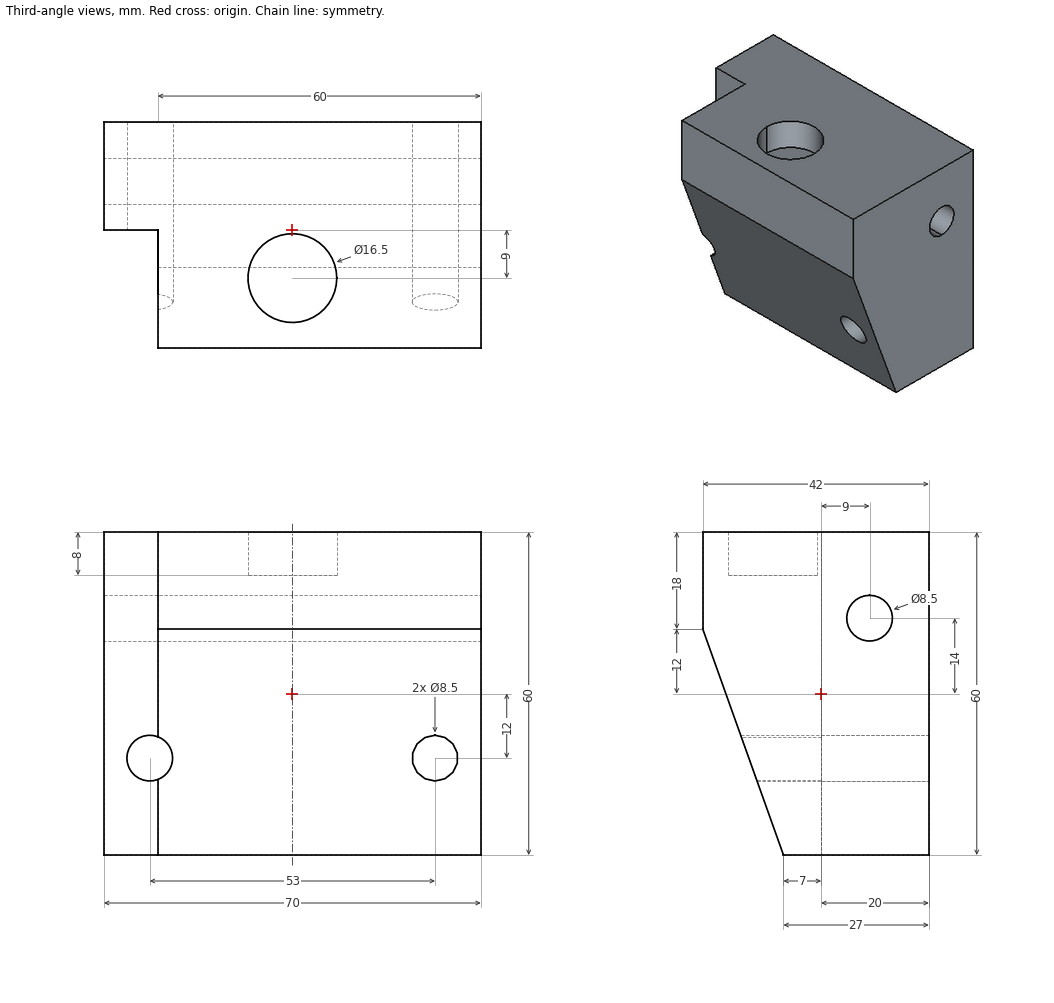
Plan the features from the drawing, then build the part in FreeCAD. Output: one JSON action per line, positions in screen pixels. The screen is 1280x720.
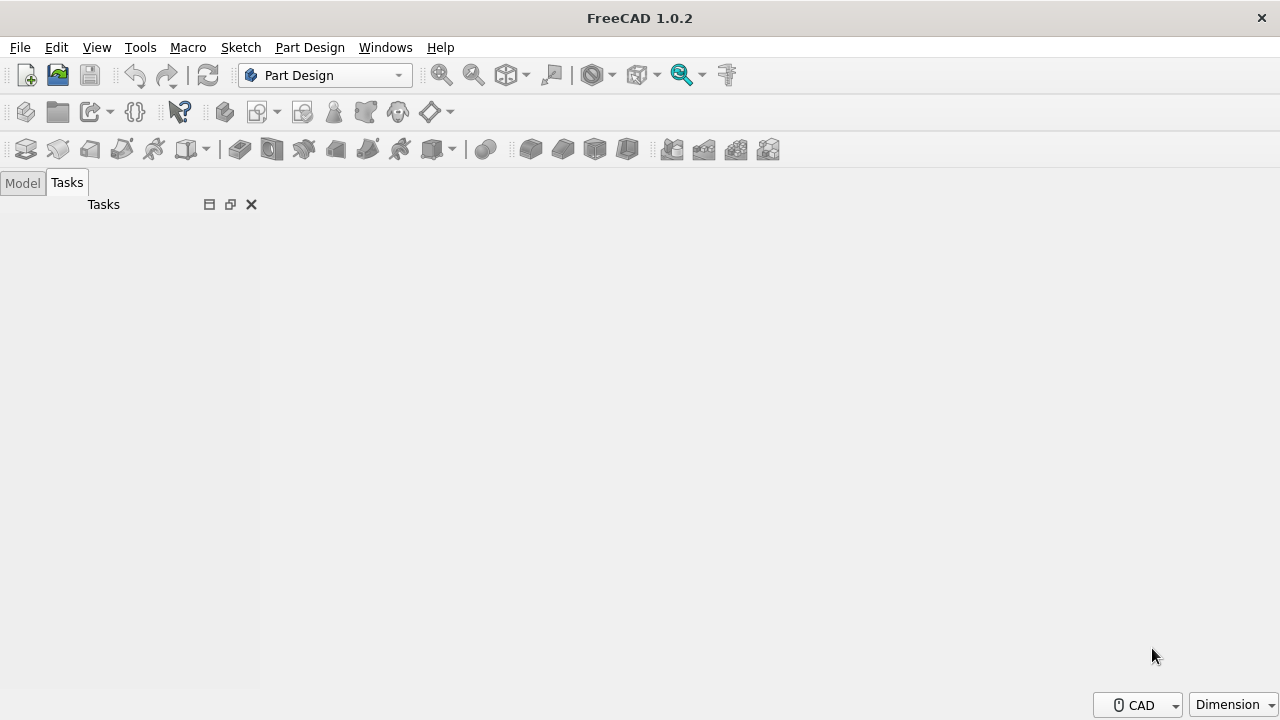
{"action": "key", "text": "ctrl+n"}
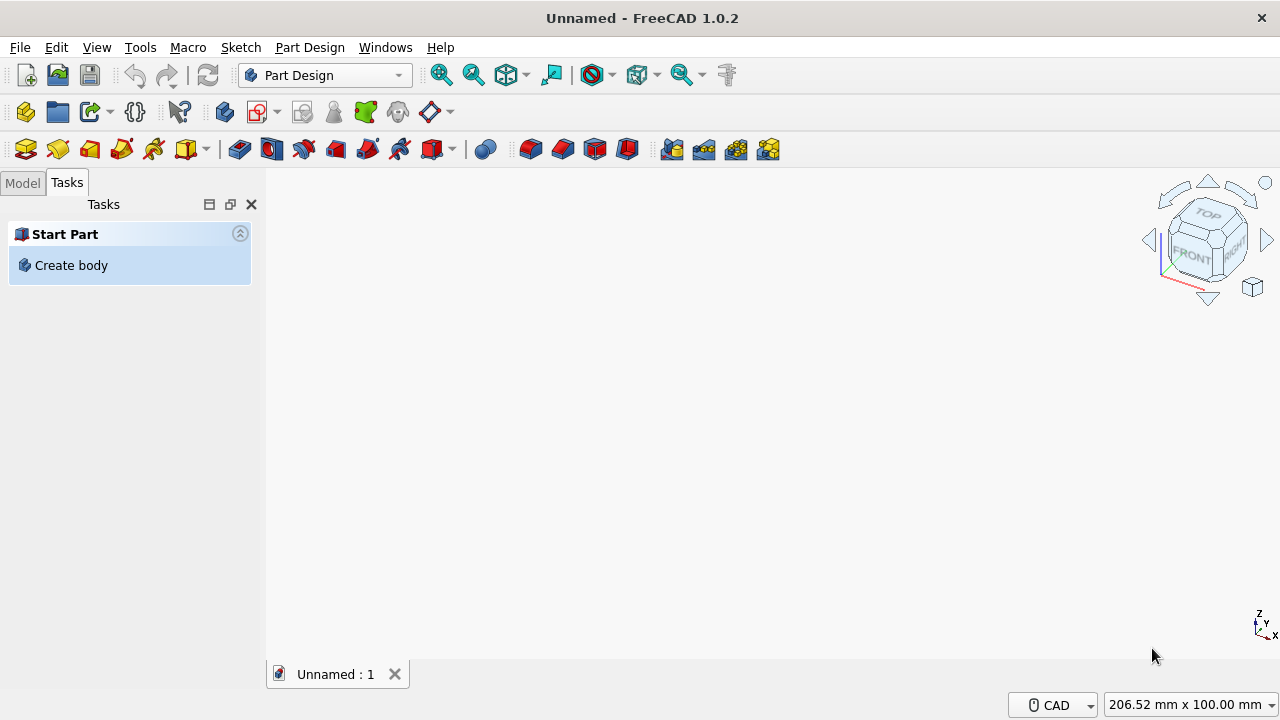
{"action": "left_click", "coordinate": [258, 112]}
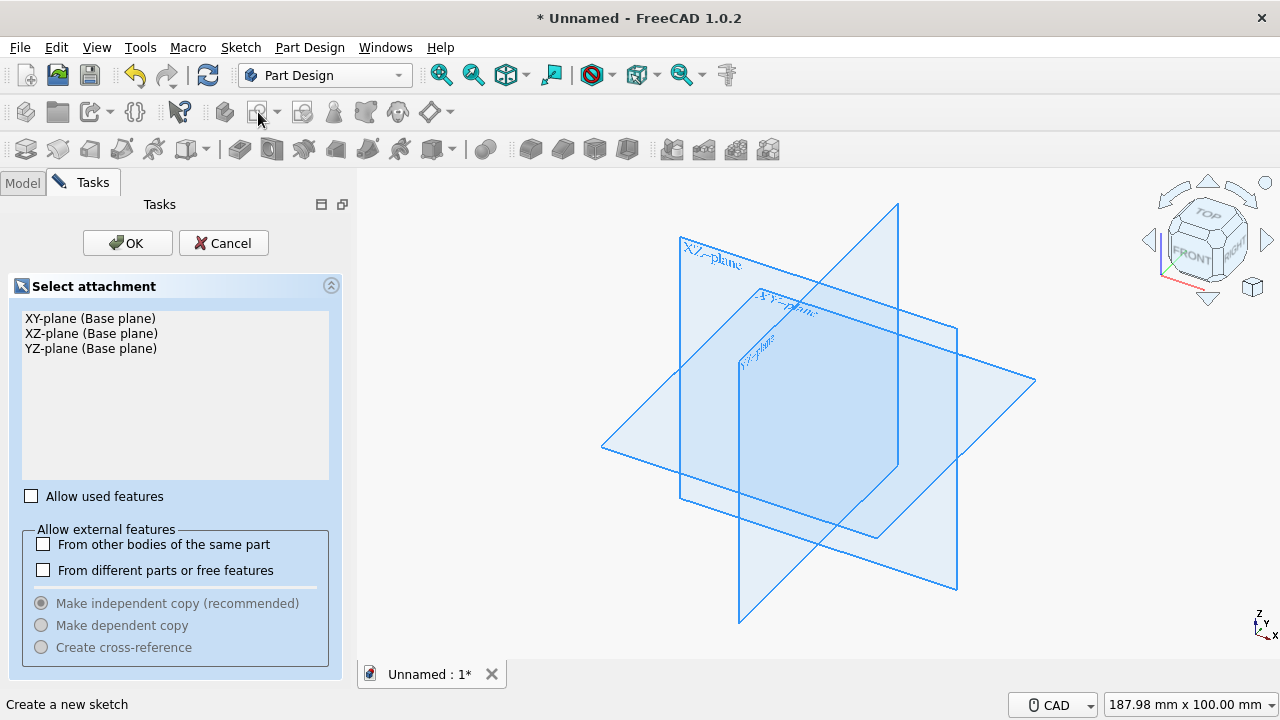
{"action": "left_click", "coordinate": [82, 334]}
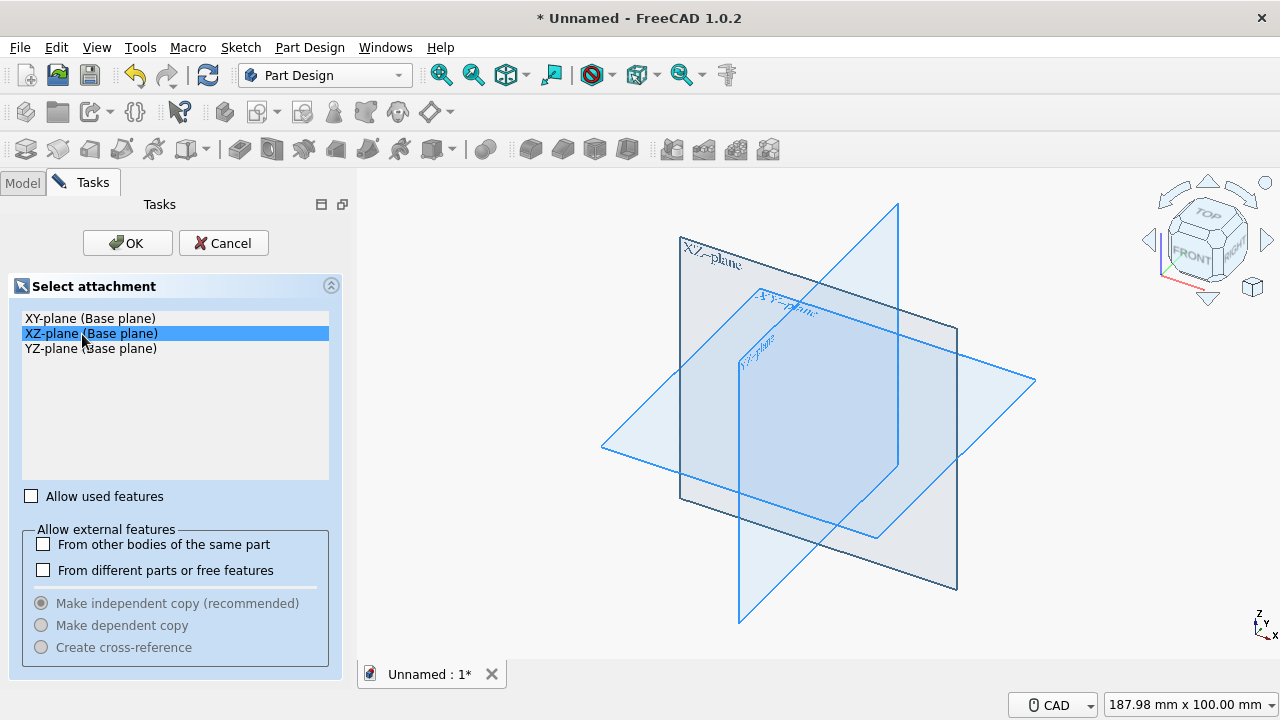
{"action": "left_click", "coordinate": [128, 243]}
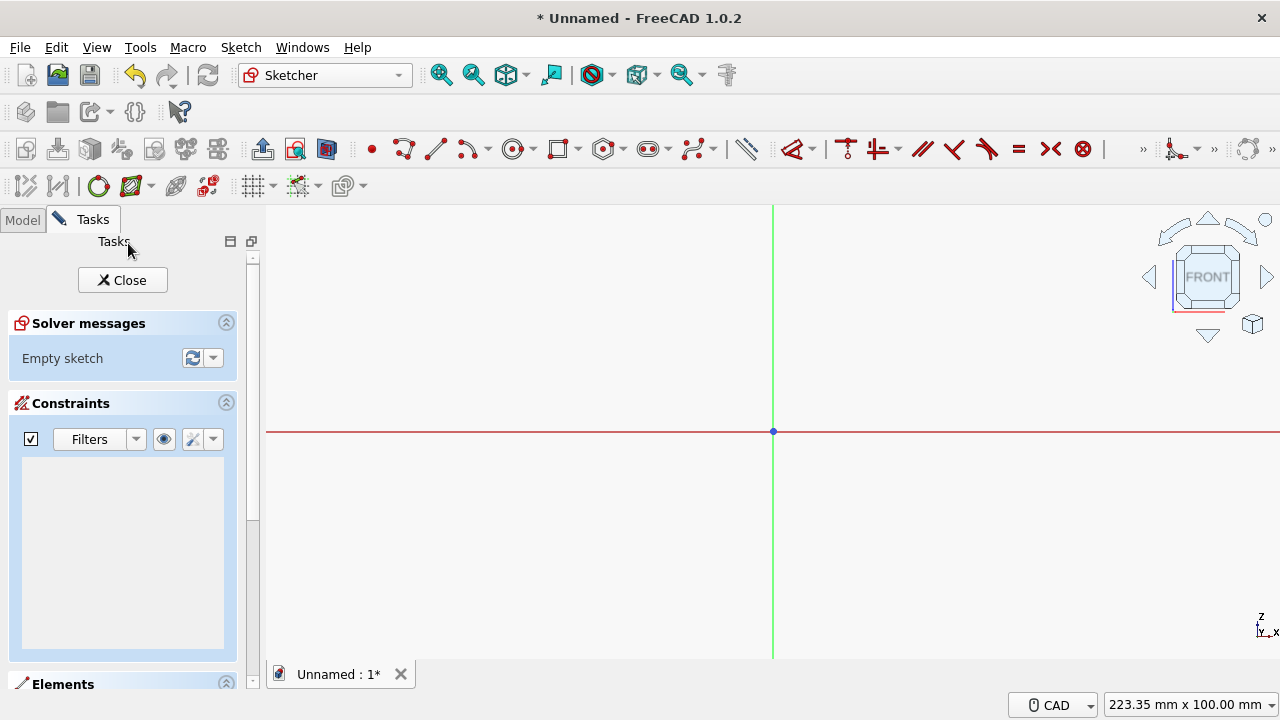
{"action": "left_click", "coordinate": [580, 150]}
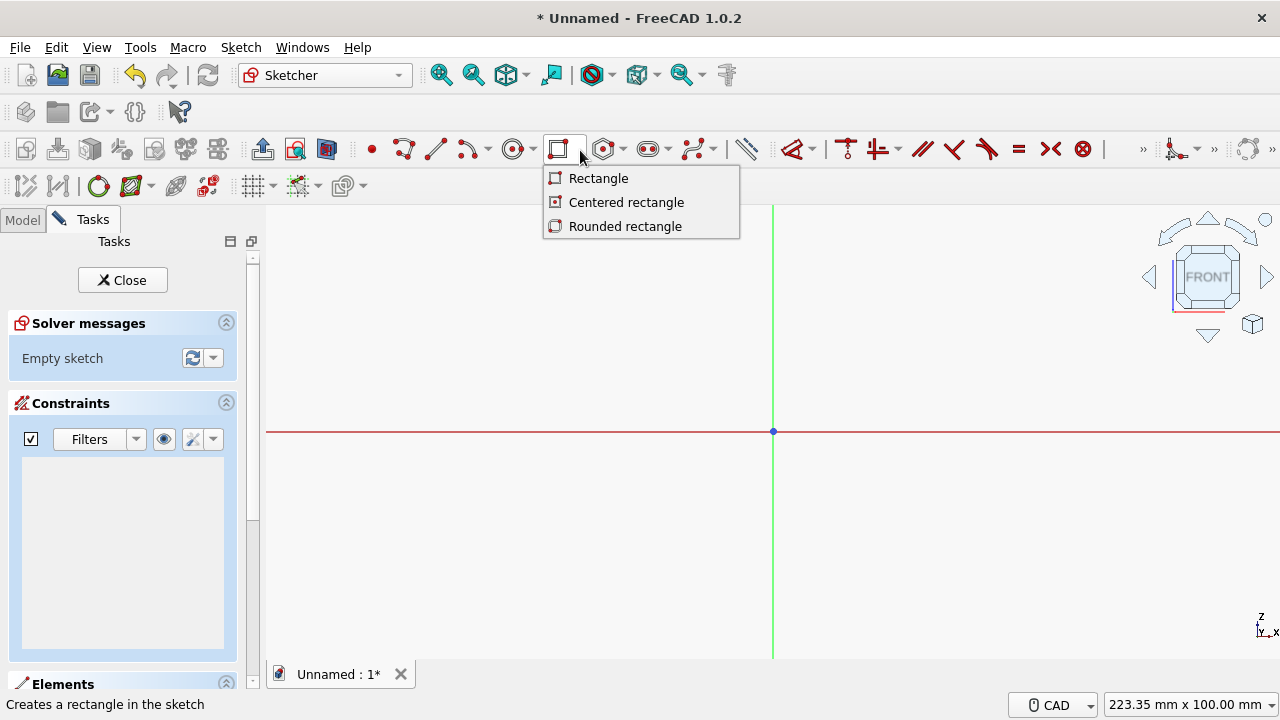
{"action": "left_click", "coordinate": [642, 202]}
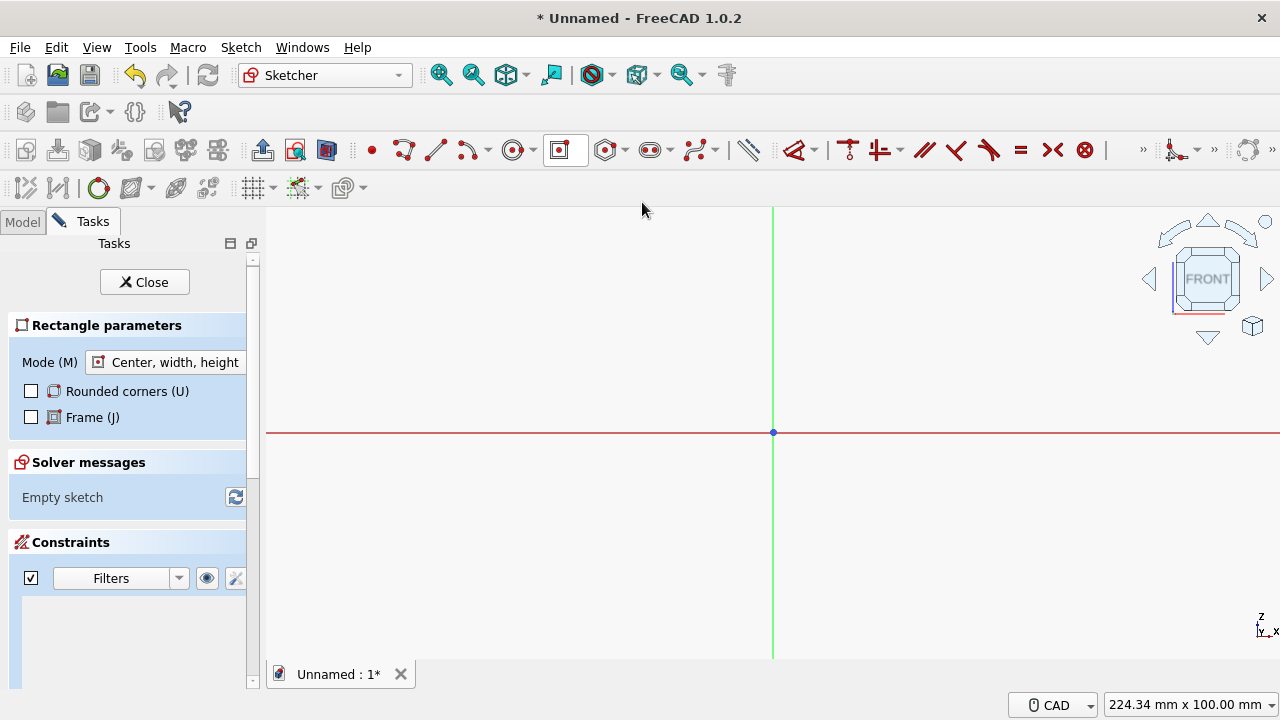
{"action": "left_click", "coordinate": [773, 433]}
{"action": "mouse_move", "coordinate": [931, 297]}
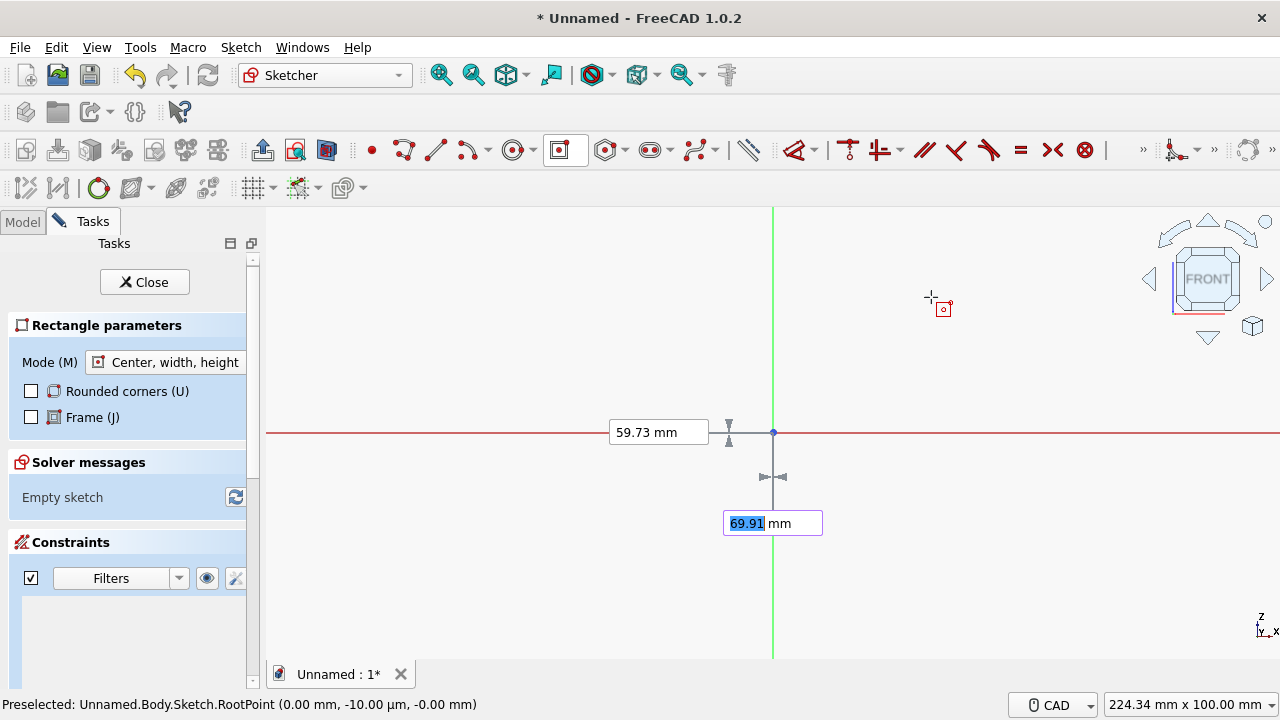
{"action": "type", "text": "70"}
{"action": "key", "text": "Tab"}
{"action": "type", "text": "60"}
{"action": "key", "text": "Return"}
{"action": "key", "text": "Escape"}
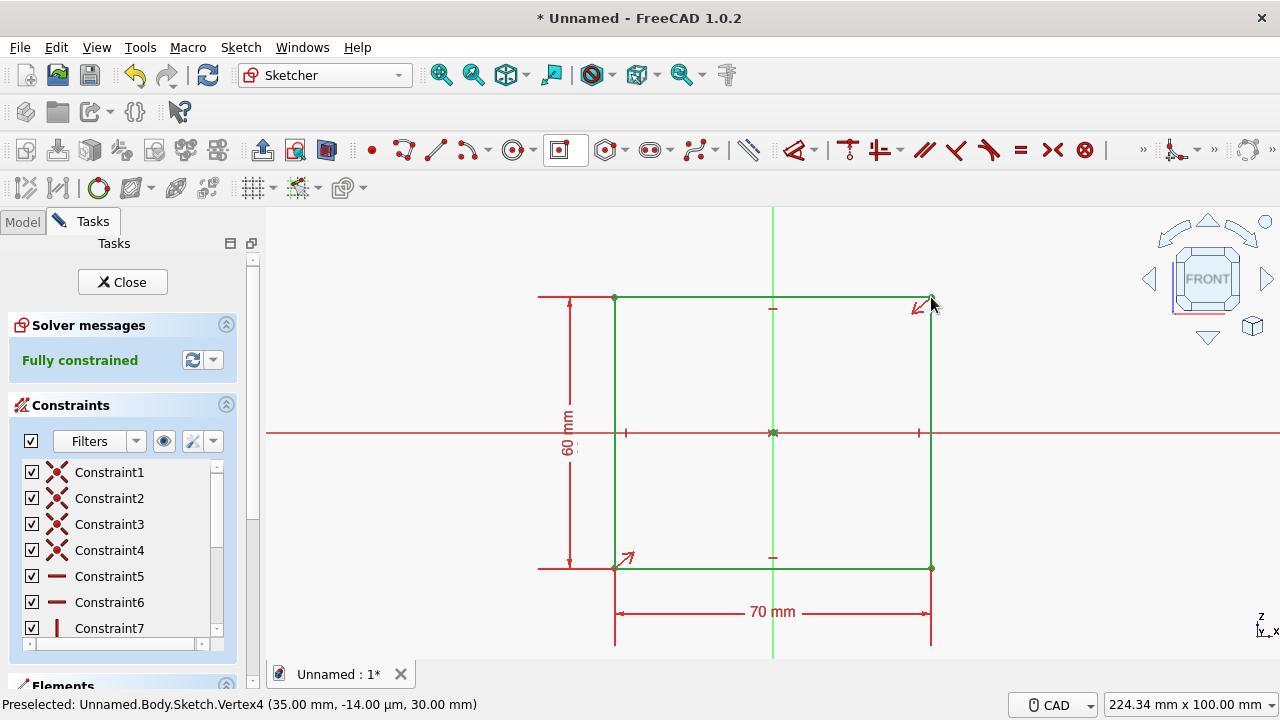
{"action": "left_click", "coordinate": [123, 282]}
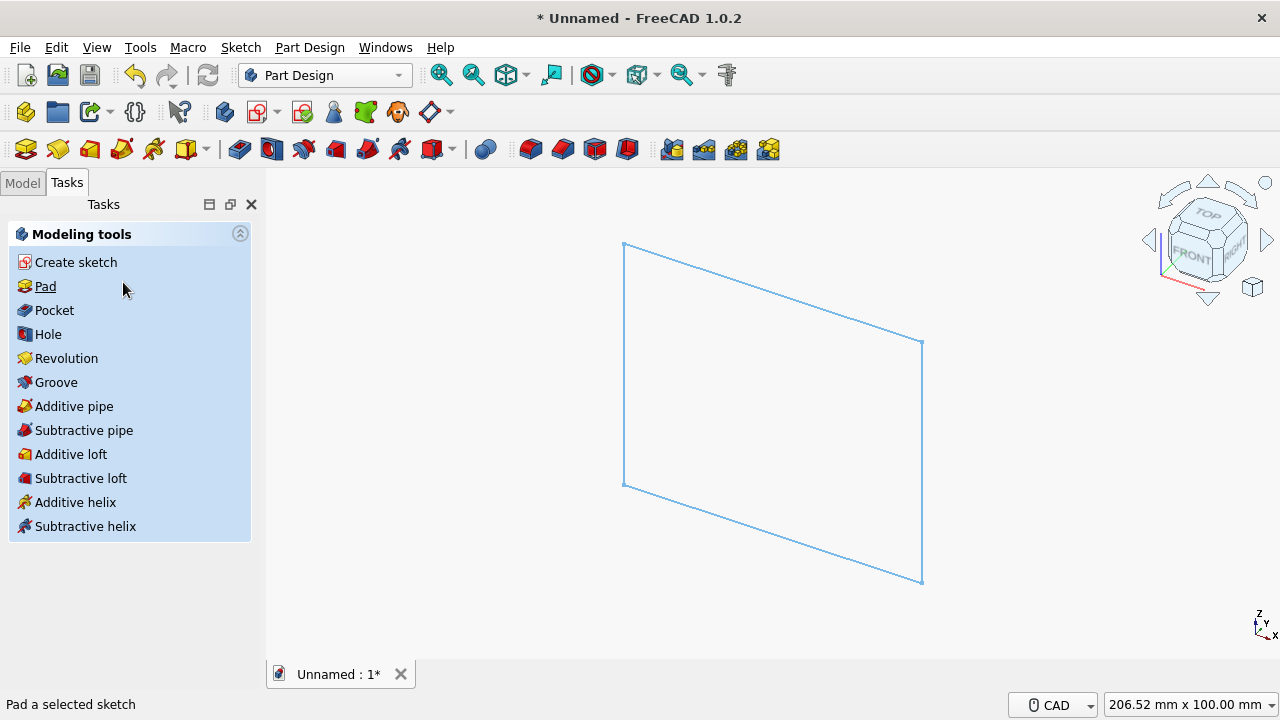
{"action": "left_click", "coordinate": [26, 150]}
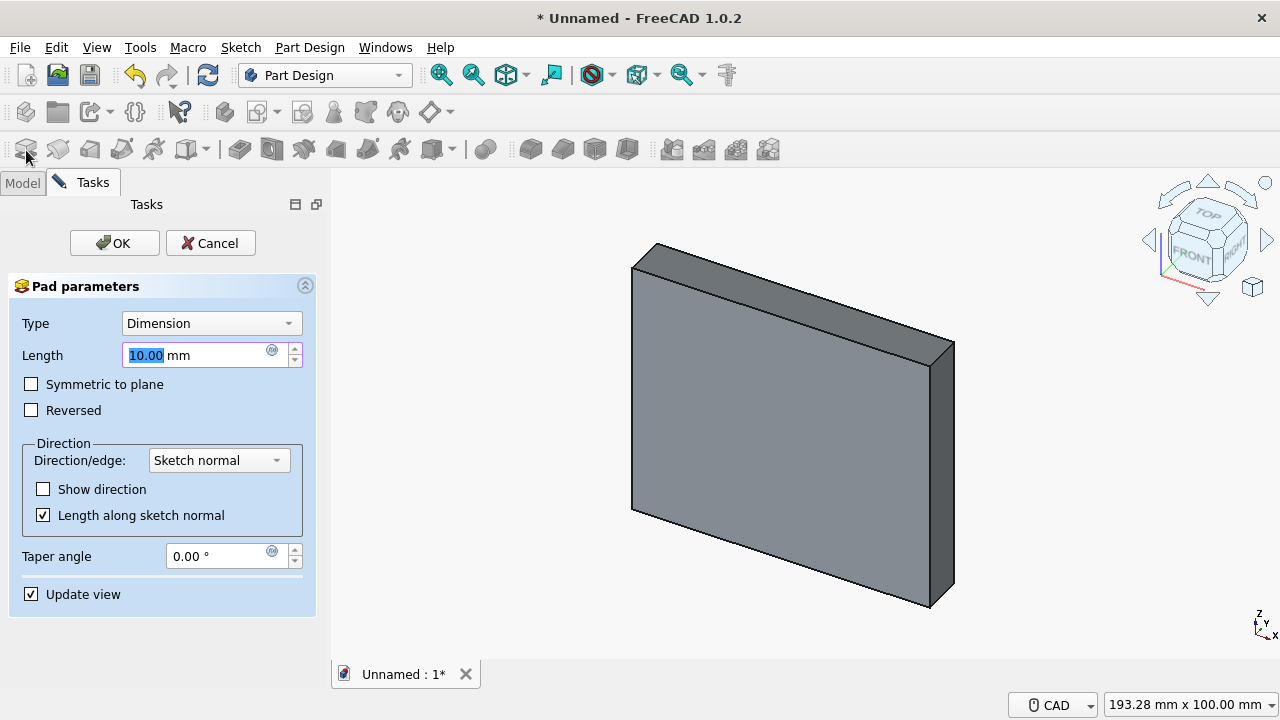
{"action": "type", "text": "20"}
{"action": "key", "text": "Tab"}